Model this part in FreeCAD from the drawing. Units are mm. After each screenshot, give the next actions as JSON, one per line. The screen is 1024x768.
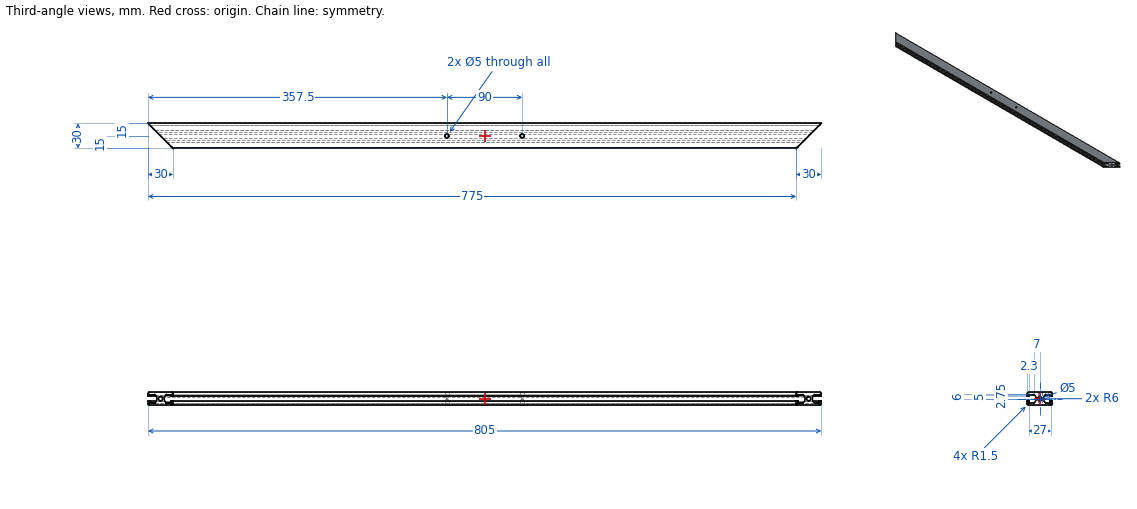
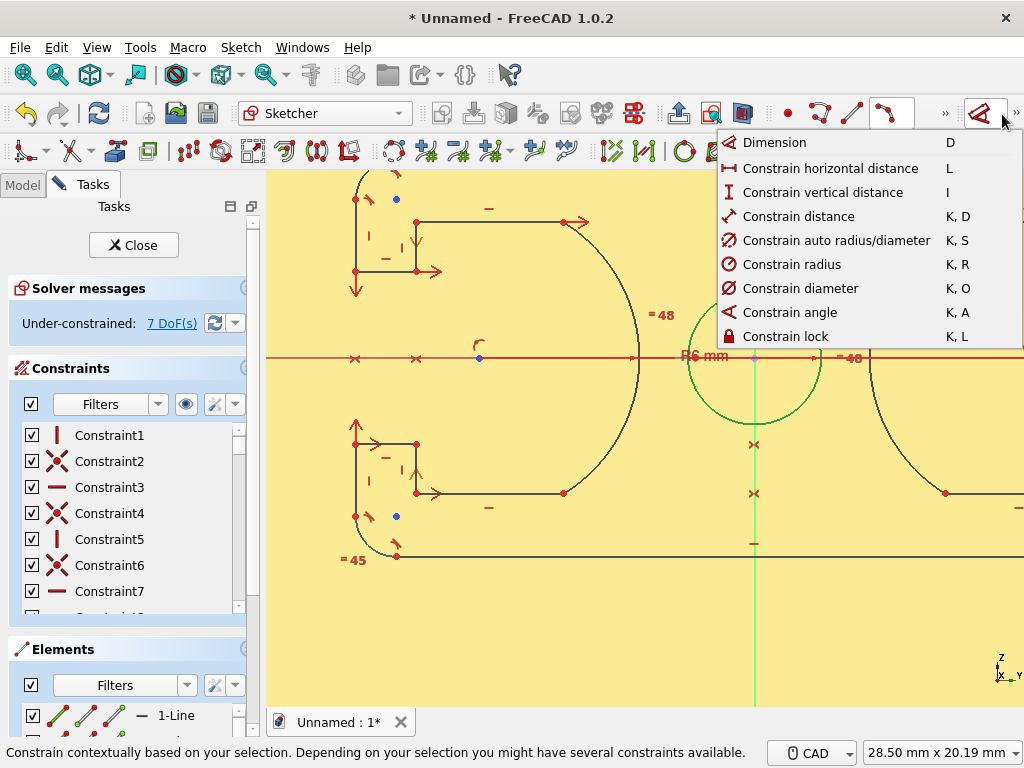
{"action": "left_click", "coordinate": [870, 264]}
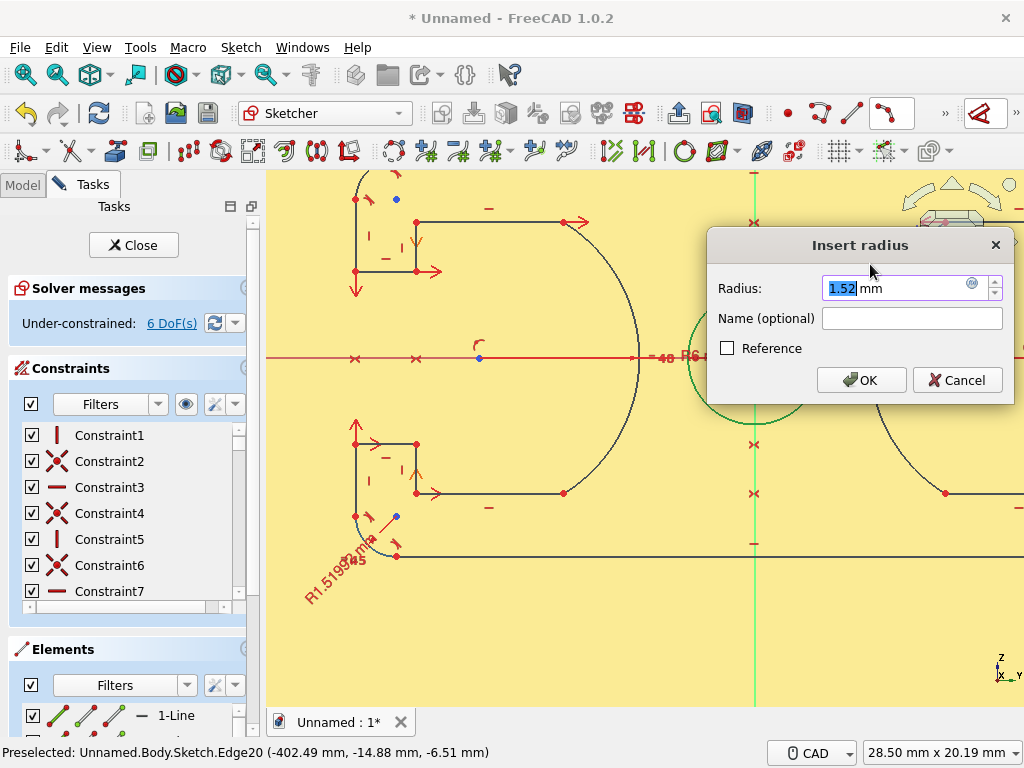
{"action": "type", "text": "1.5"}
{"action": "key", "text": "Return"}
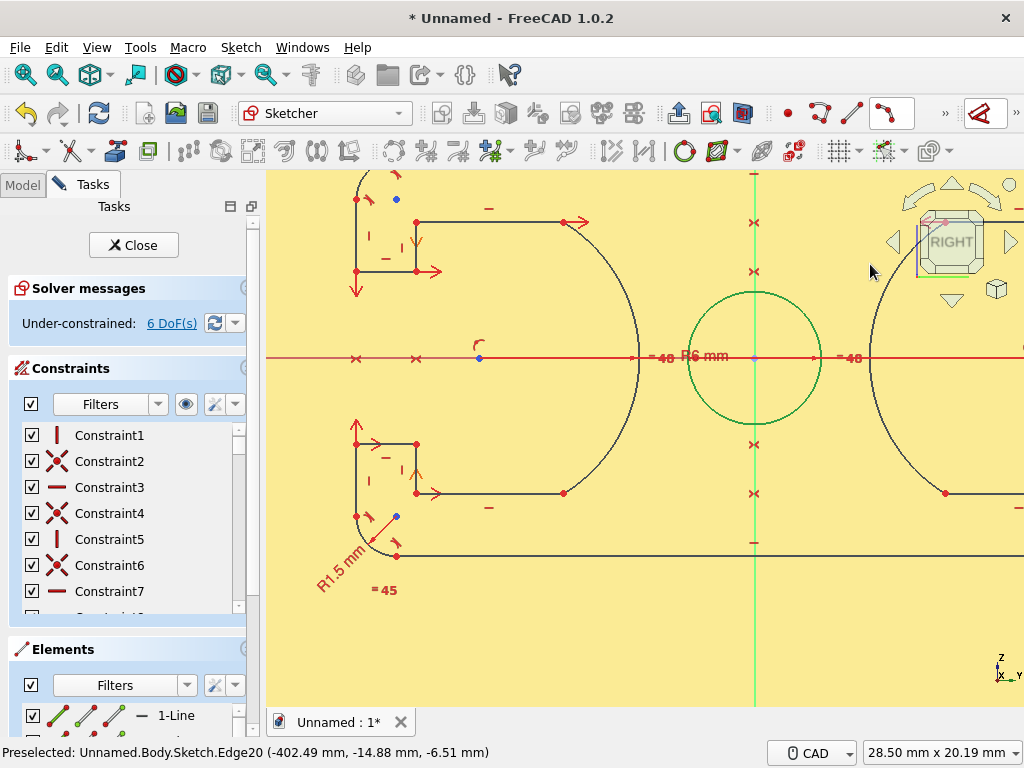
{"action": "left_click", "coordinate": [611, 556]}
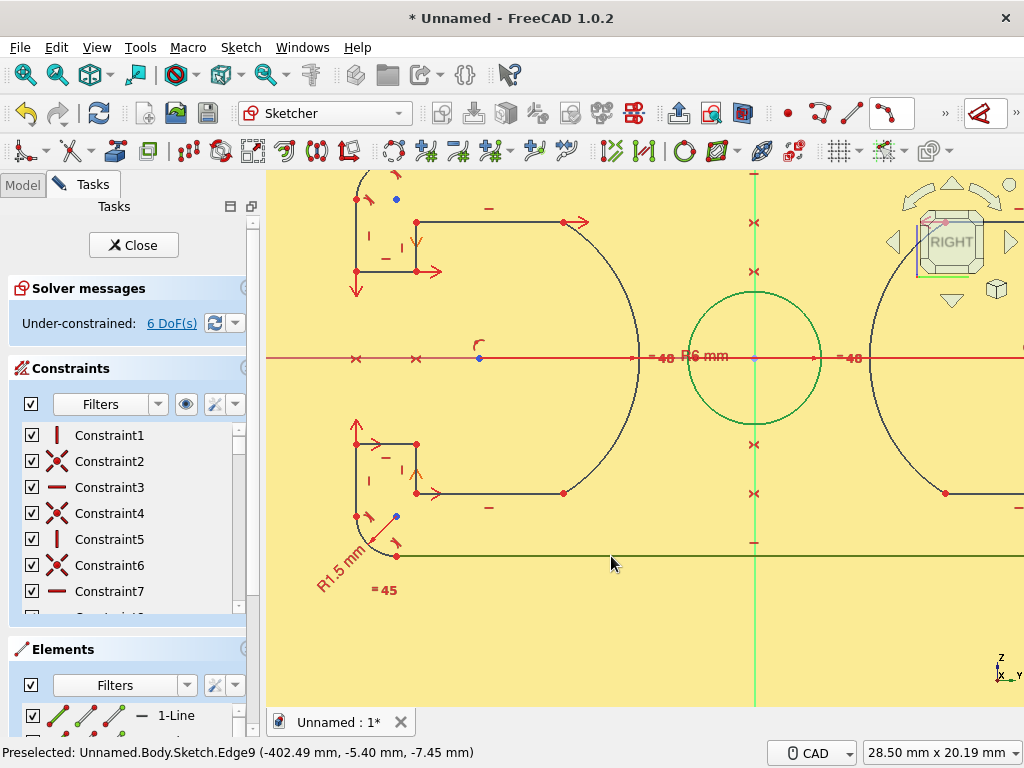
{"action": "left_click", "coordinate": [1002, 114]}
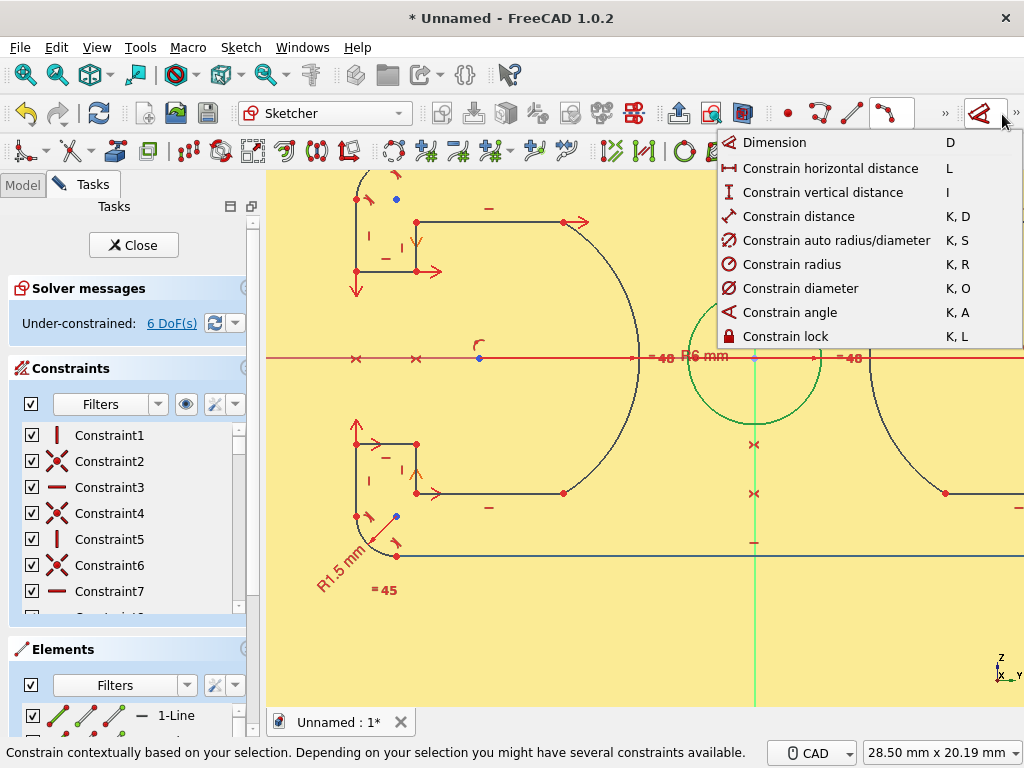
{"action": "left_click", "coordinate": [870, 168]}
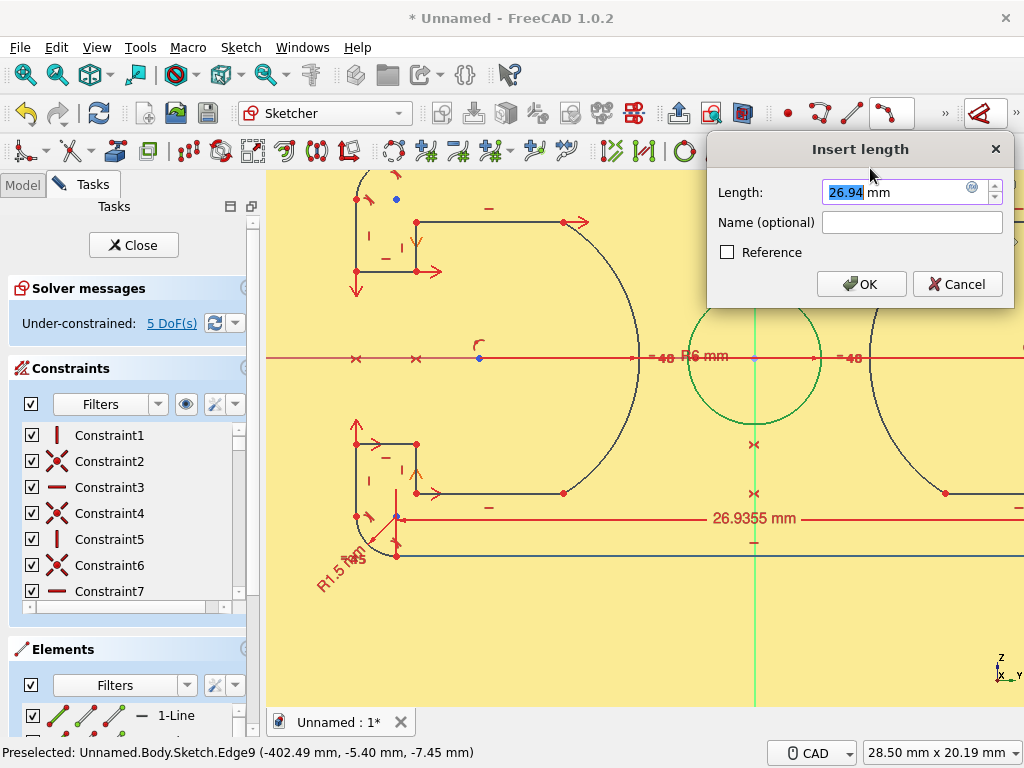
{"action": "type", "text": "27"}
{"action": "key", "text": "Return"}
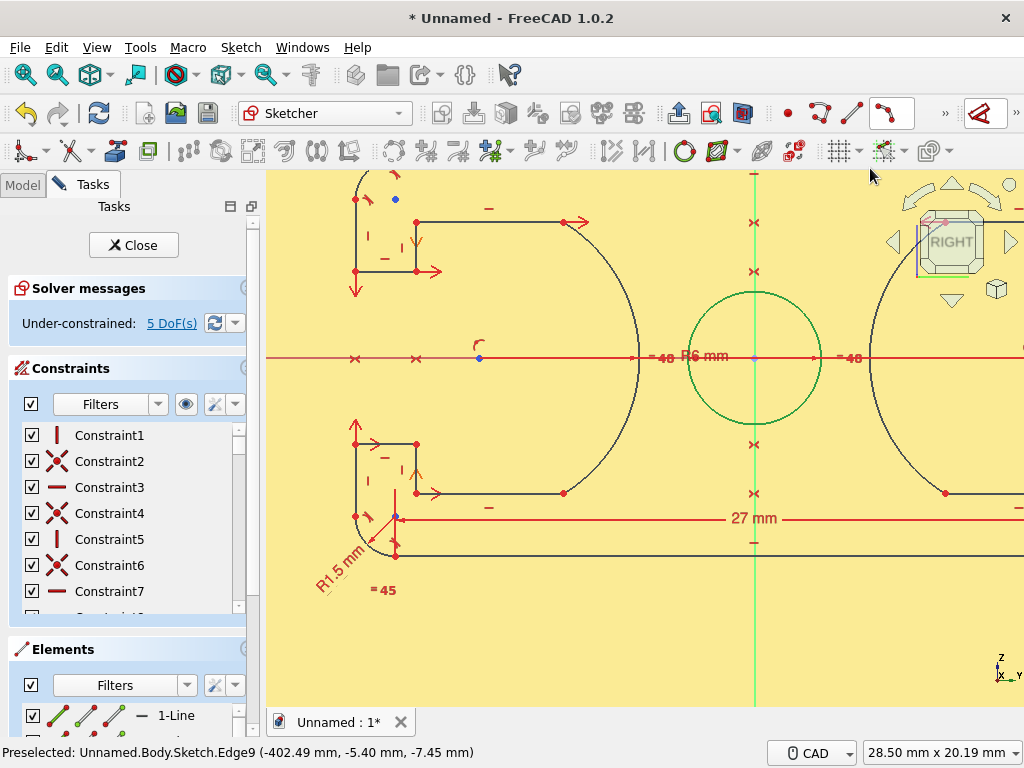
{"action": "left_click", "coordinate": [356, 200]}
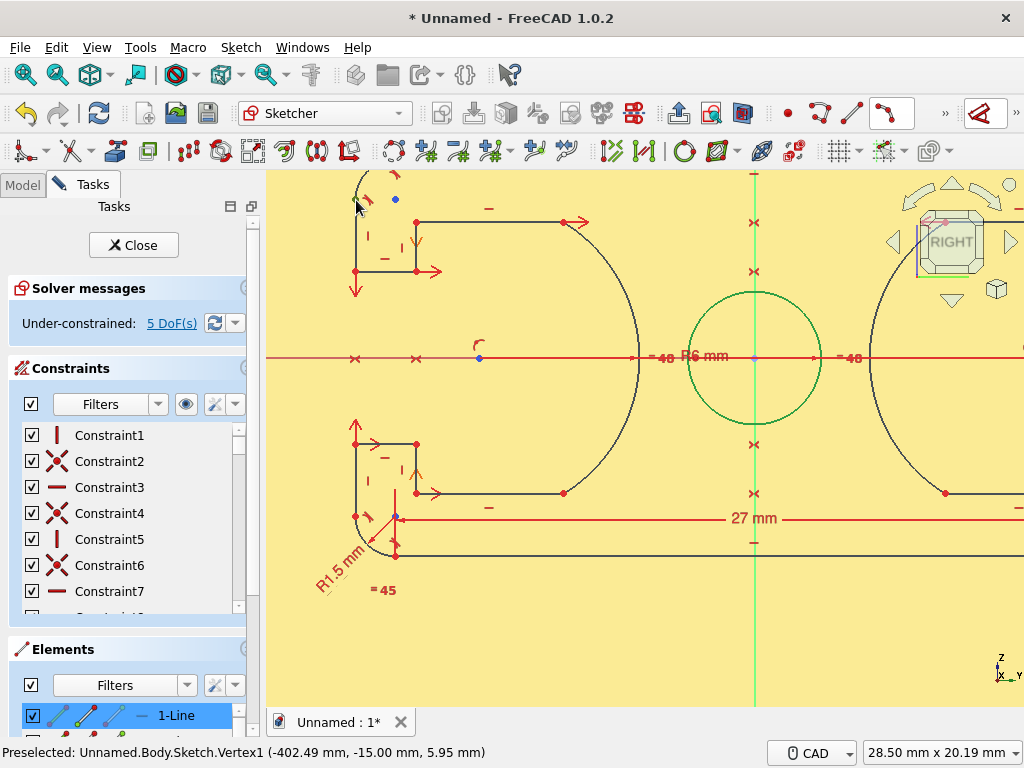
{"action": "left_click", "coordinate": [1002, 114]}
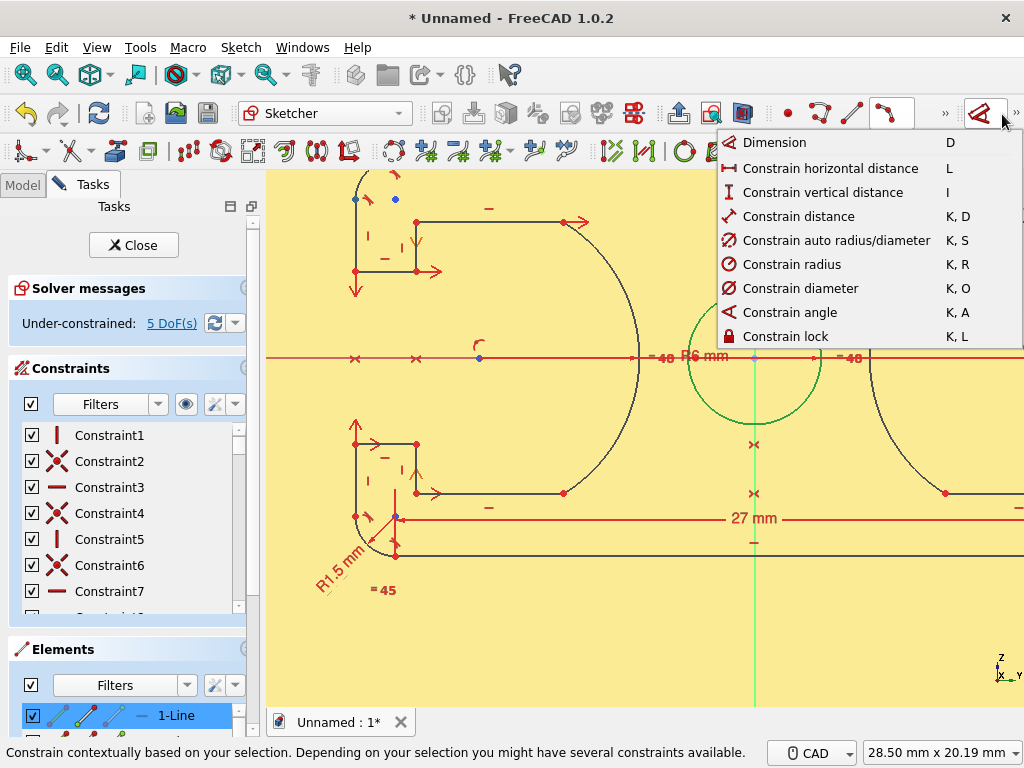
{"action": "left_click", "coordinate": [870, 192]}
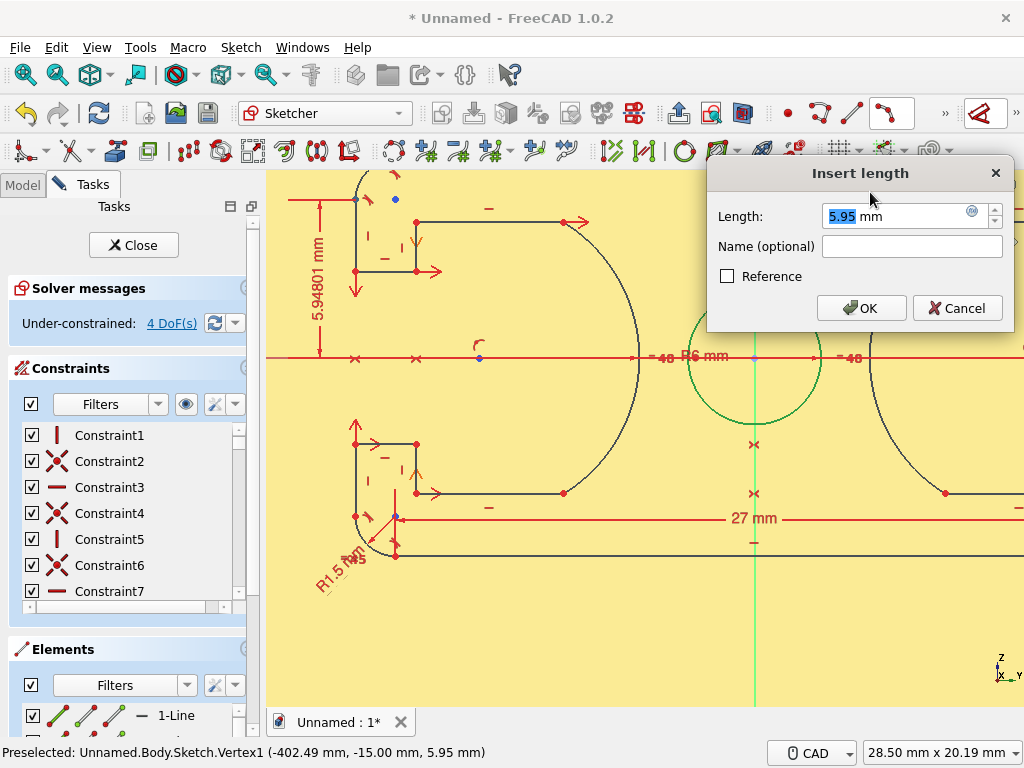
{"action": "type", "text": "6"}
{"action": "key", "text": "Return"}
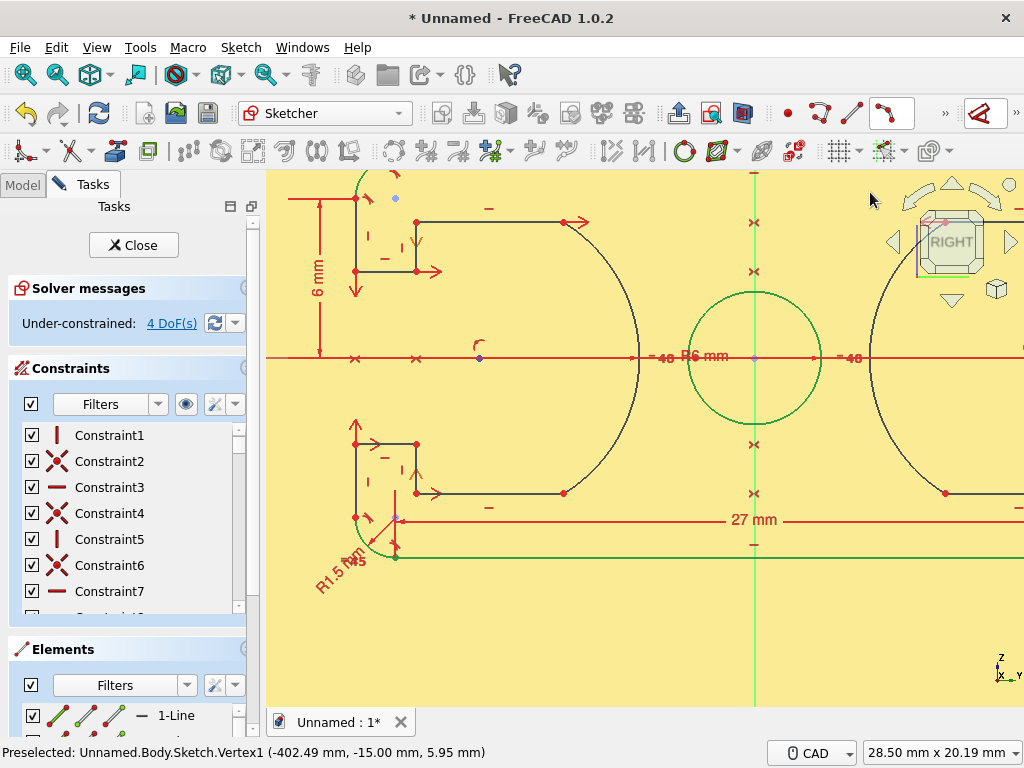
{"action": "left_click", "coordinate": [416, 222]}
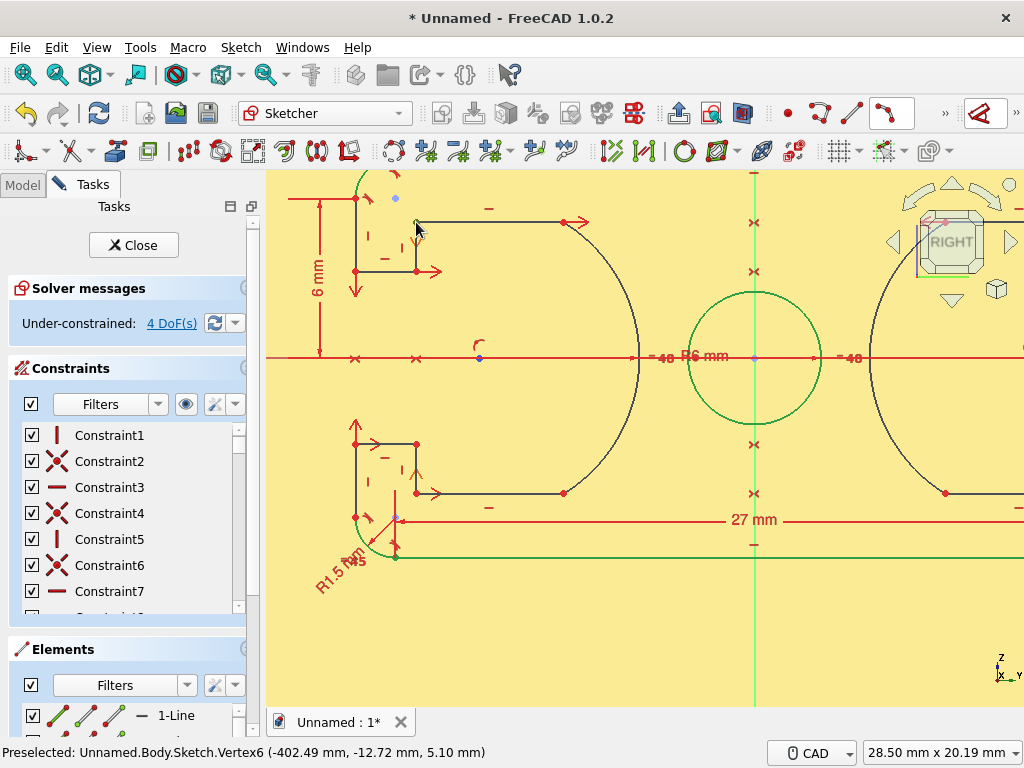
{"action": "left_click", "coordinate": [1002, 114]}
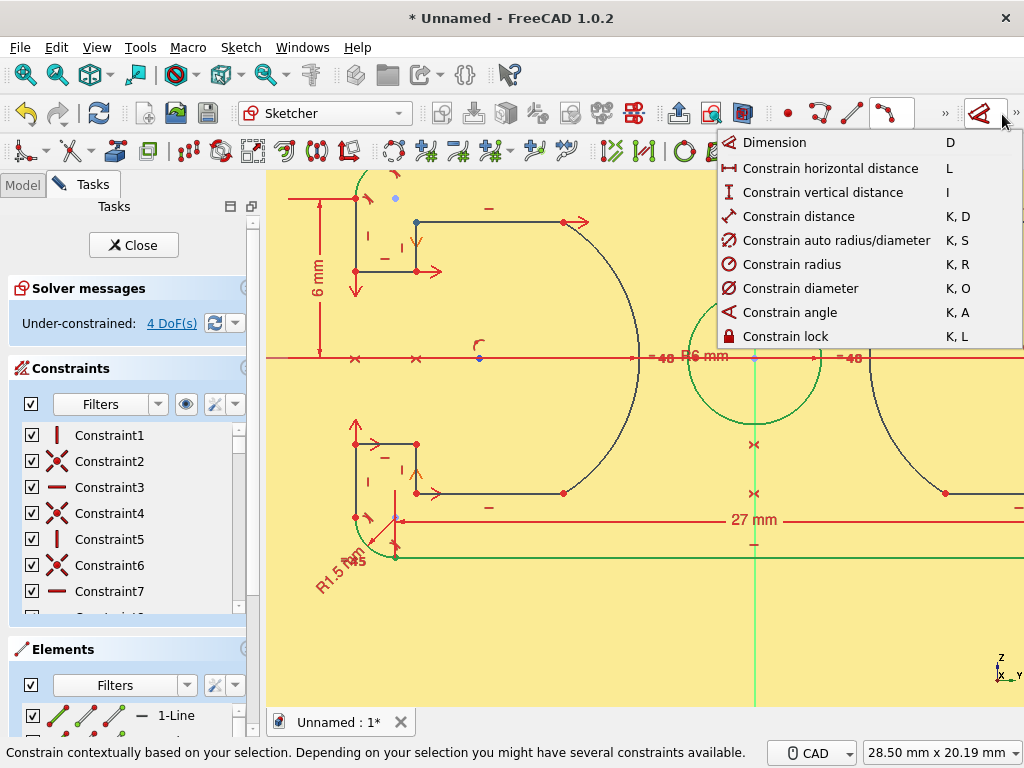
{"action": "left_click", "coordinate": [870, 192]}